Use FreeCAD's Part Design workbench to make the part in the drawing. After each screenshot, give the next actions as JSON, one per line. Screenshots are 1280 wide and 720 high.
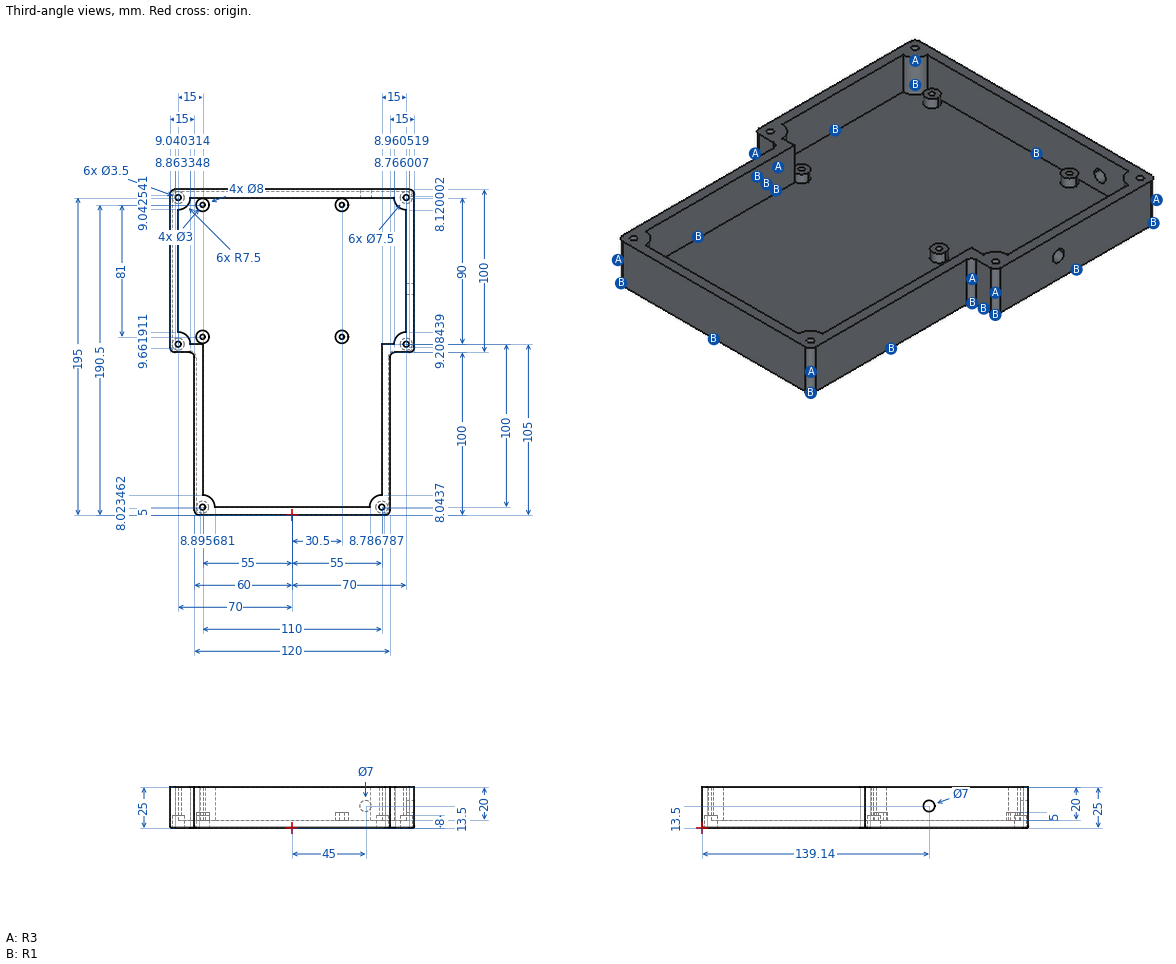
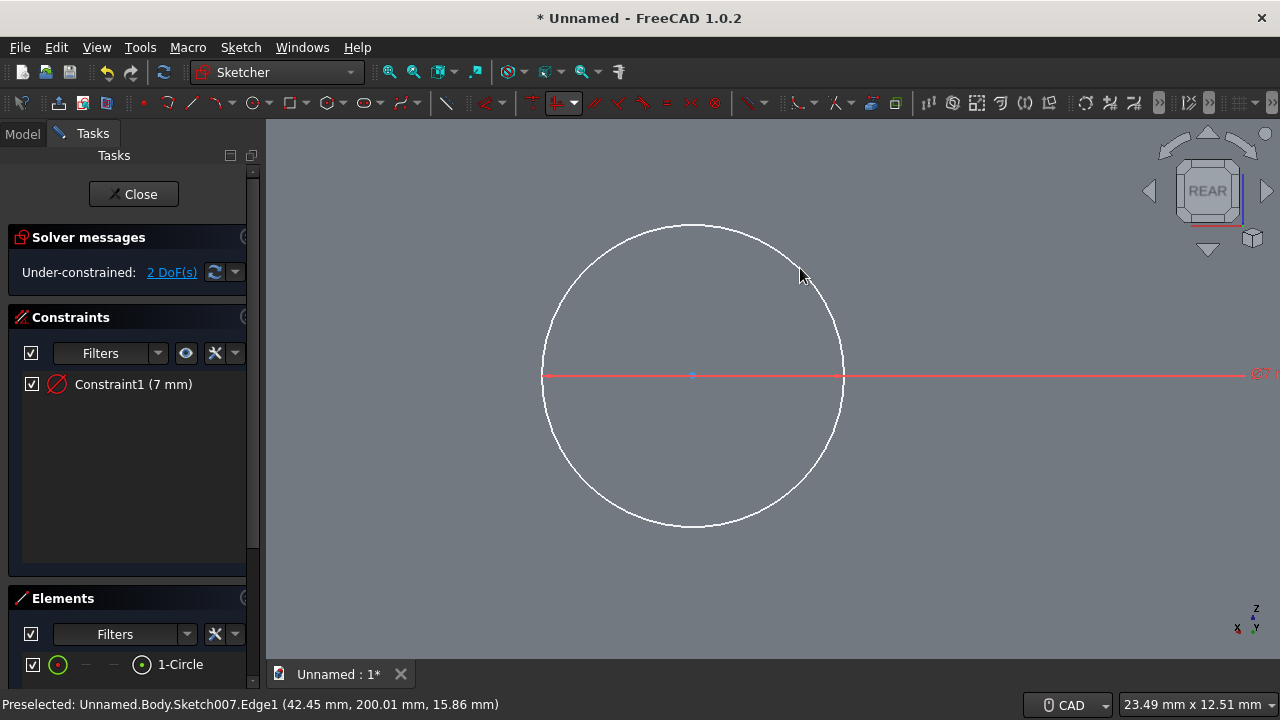
{"action": "key", "text": "d"}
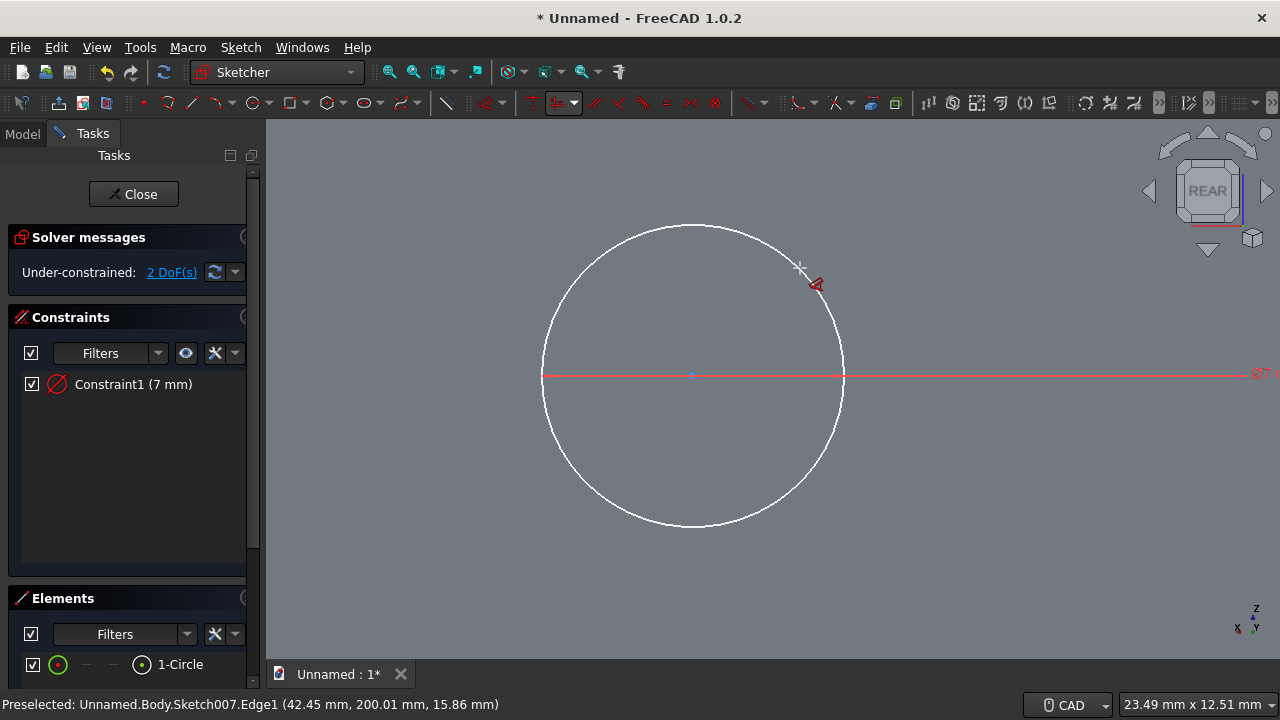
{"action": "left_click", "coordinate": [693, 376]}
{"action": "left_click", "coordinate": [904, 342]}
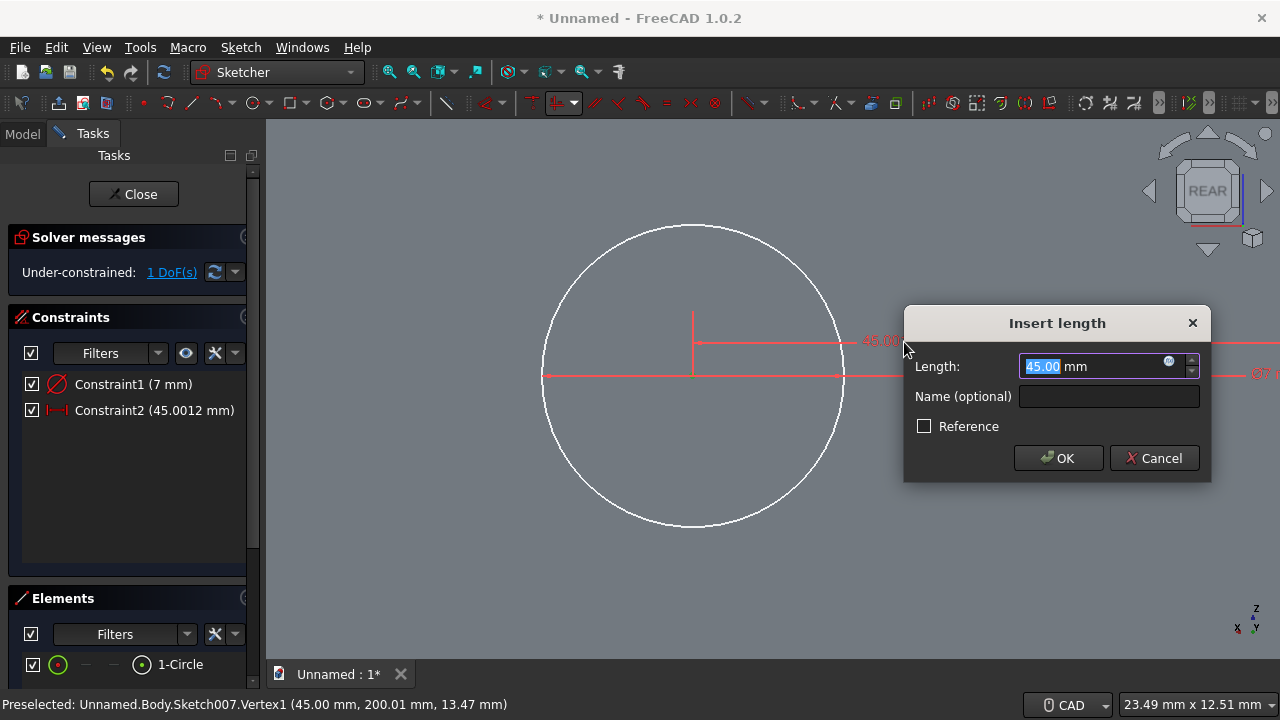
{"action": "type", "text": "45"}
{"action": "key", "text": "Return"}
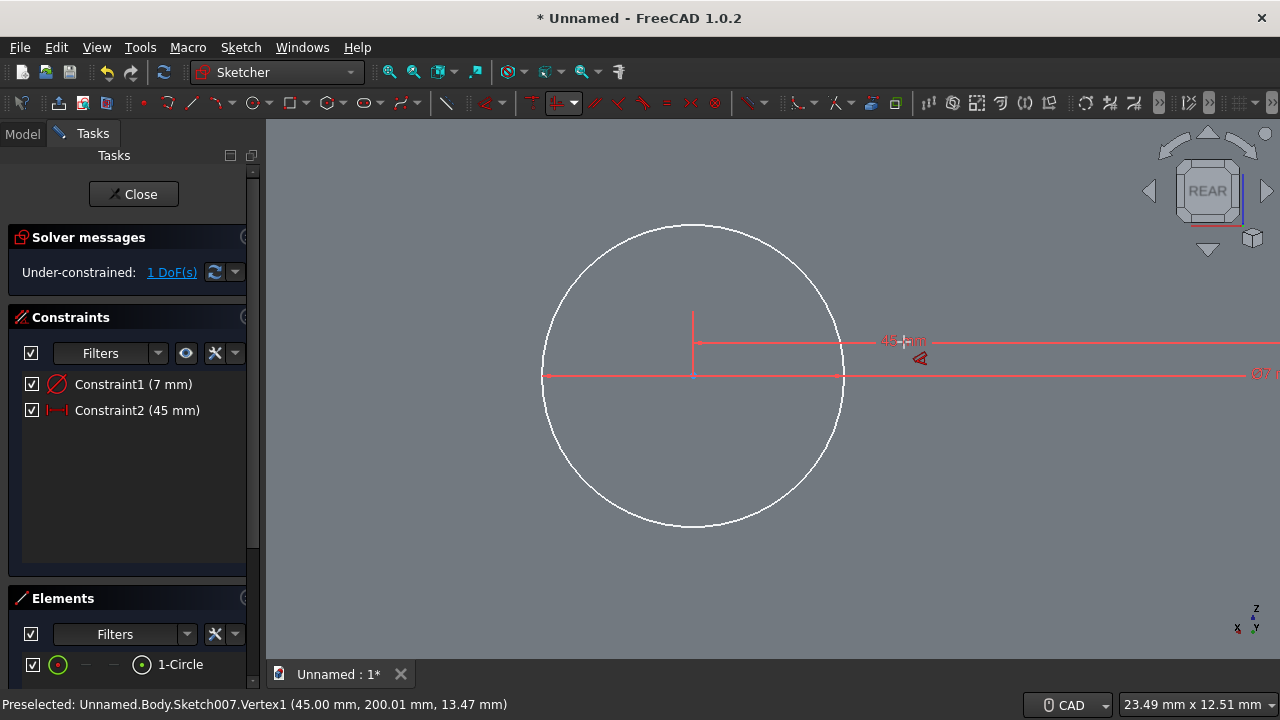
{"action": "left_click", "coordinate": [693, 376]}
{"action": "left_click", "coordinate": [659, 503]}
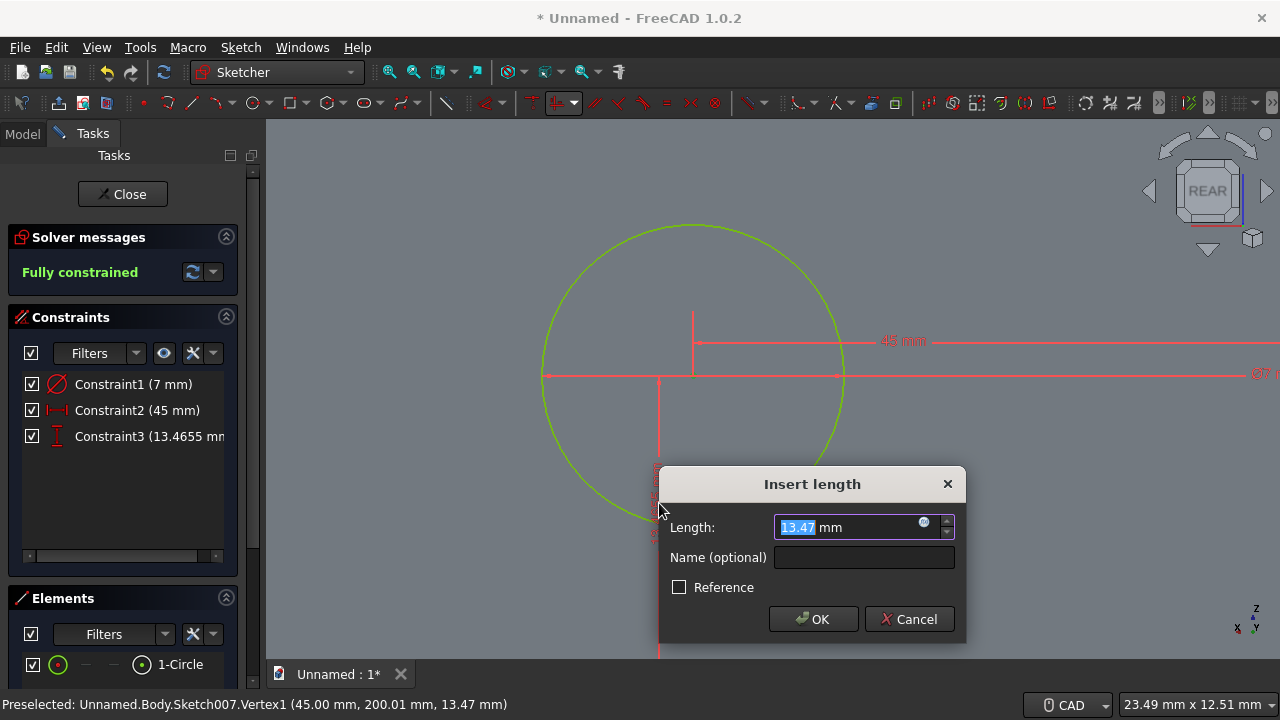
{"action": "type", "text": "13.5"}
{"action": "key", "text": "Return"}
{"action": "key", "text": "Escape"}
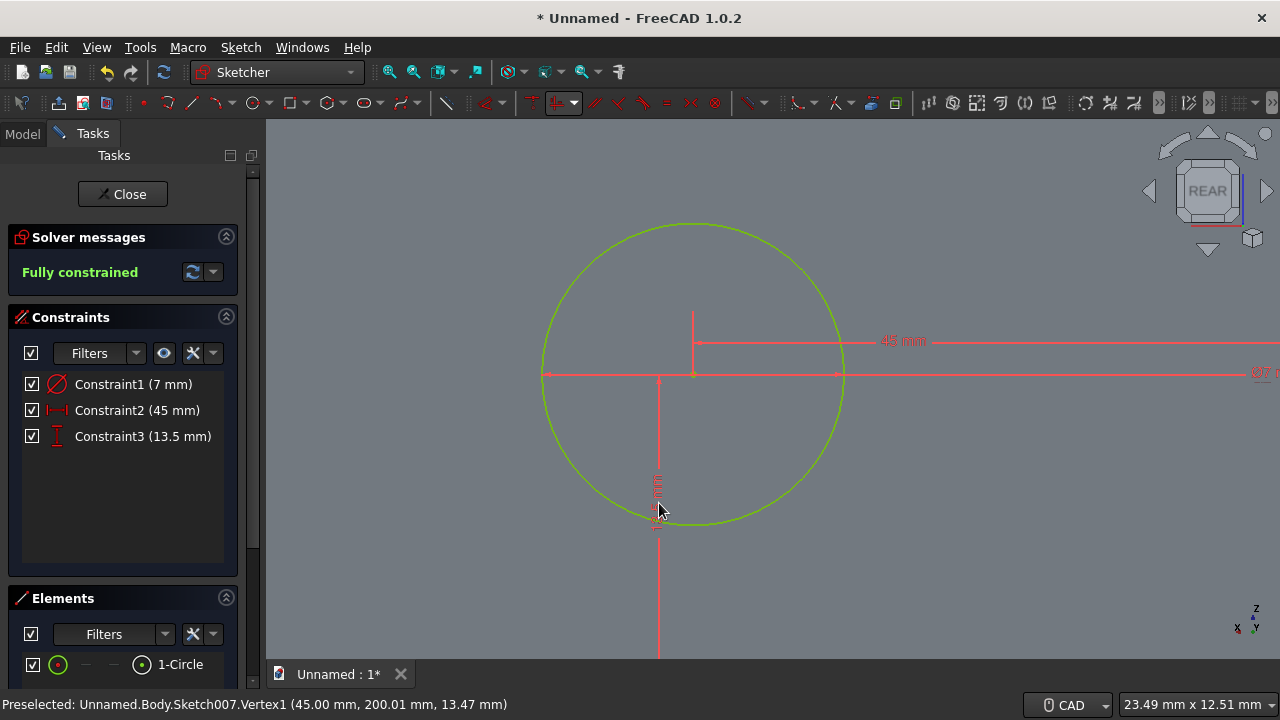
{"action": "left_click", "coordinate": [123, 194]}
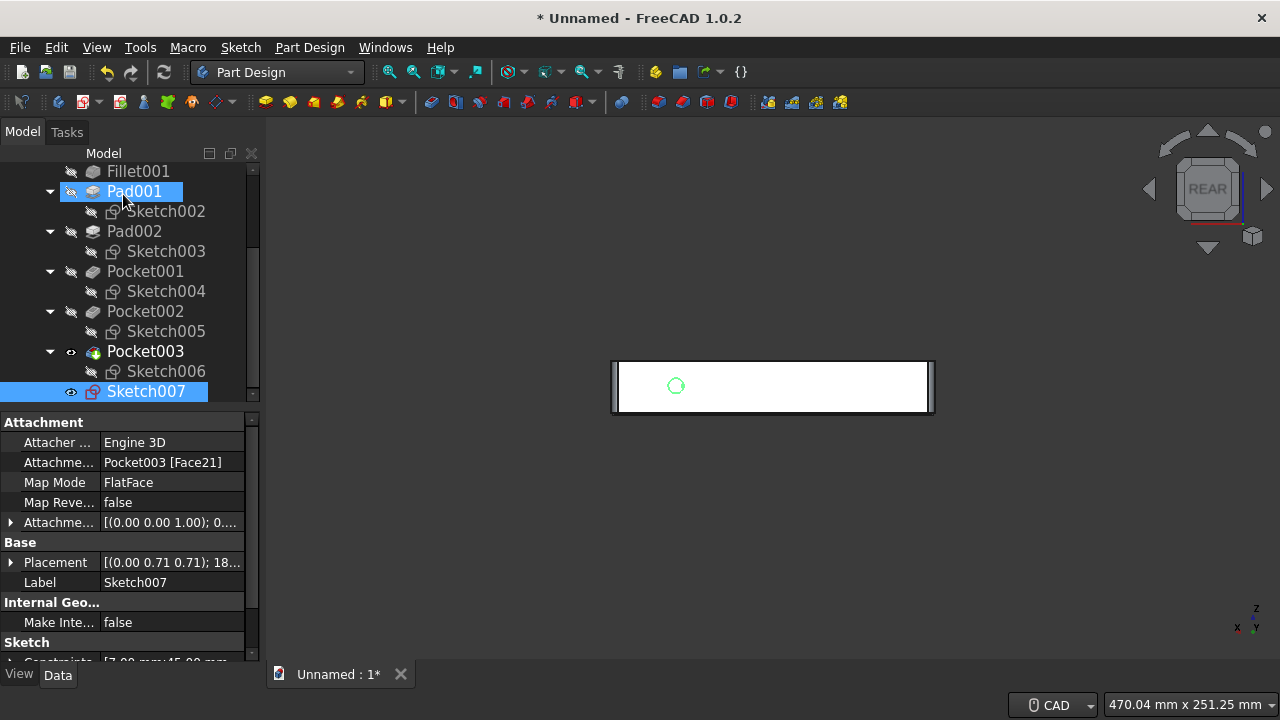
{"action": "left_click", "coordinate": [432, 102]}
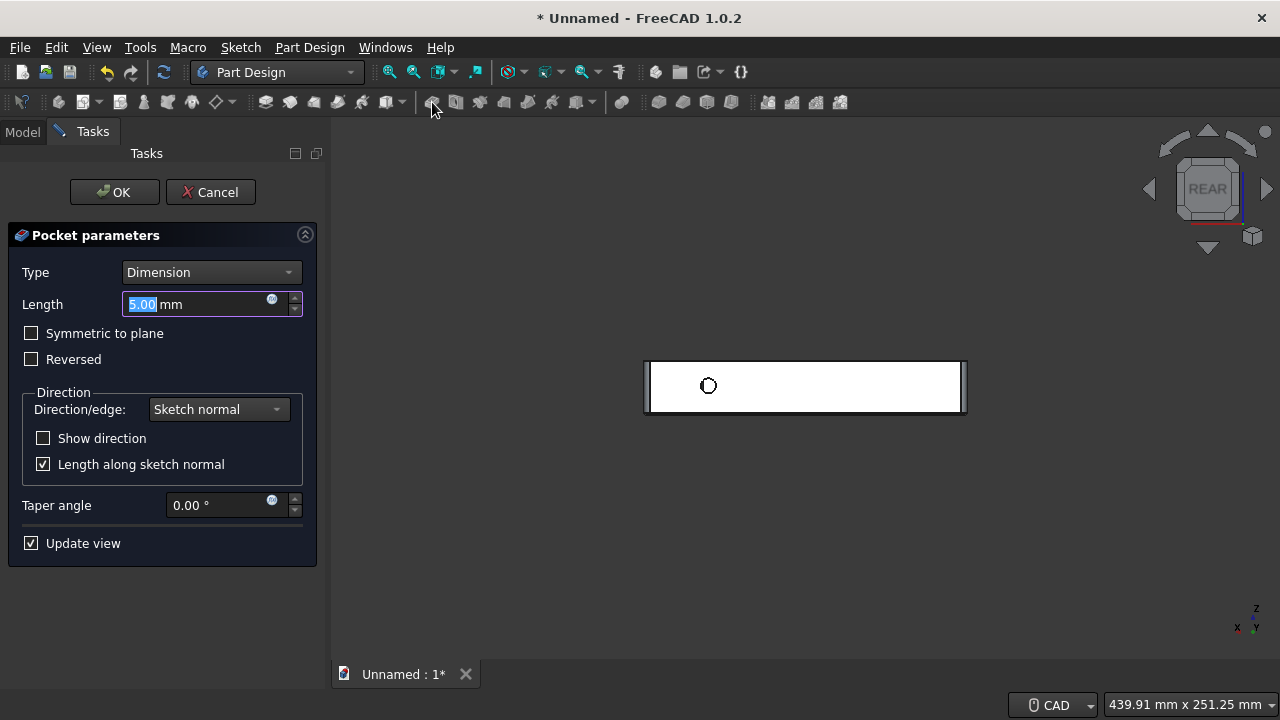
{"action": "left_click", "coordinate": [212, 272]}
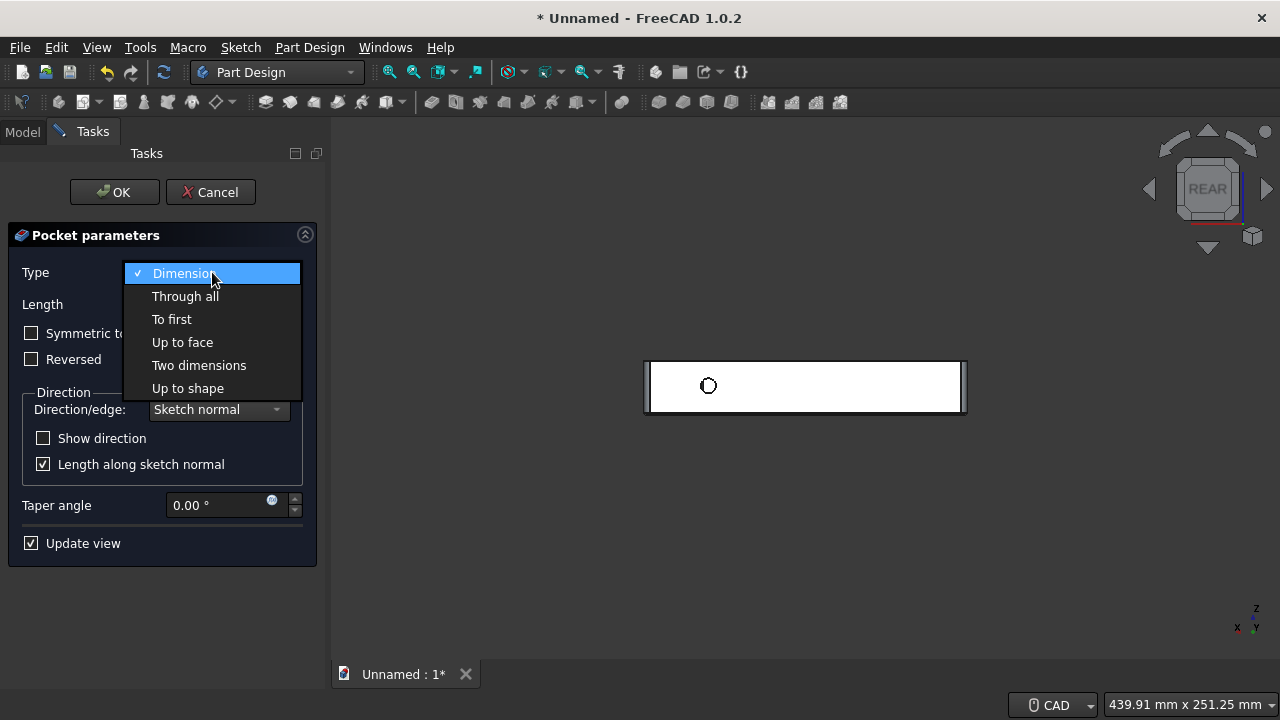
{"action": "left_click", "coordinate": [212, 320]}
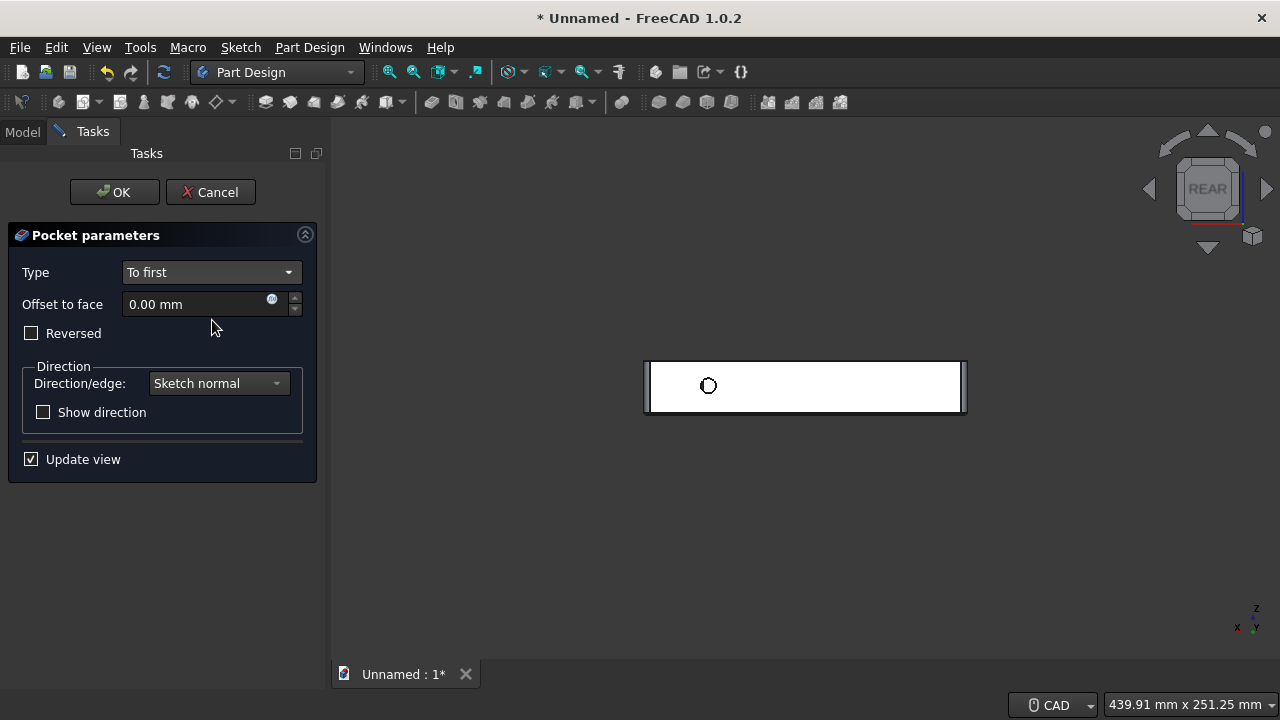
{"action": "left_click", "coordinate": [115, 192]}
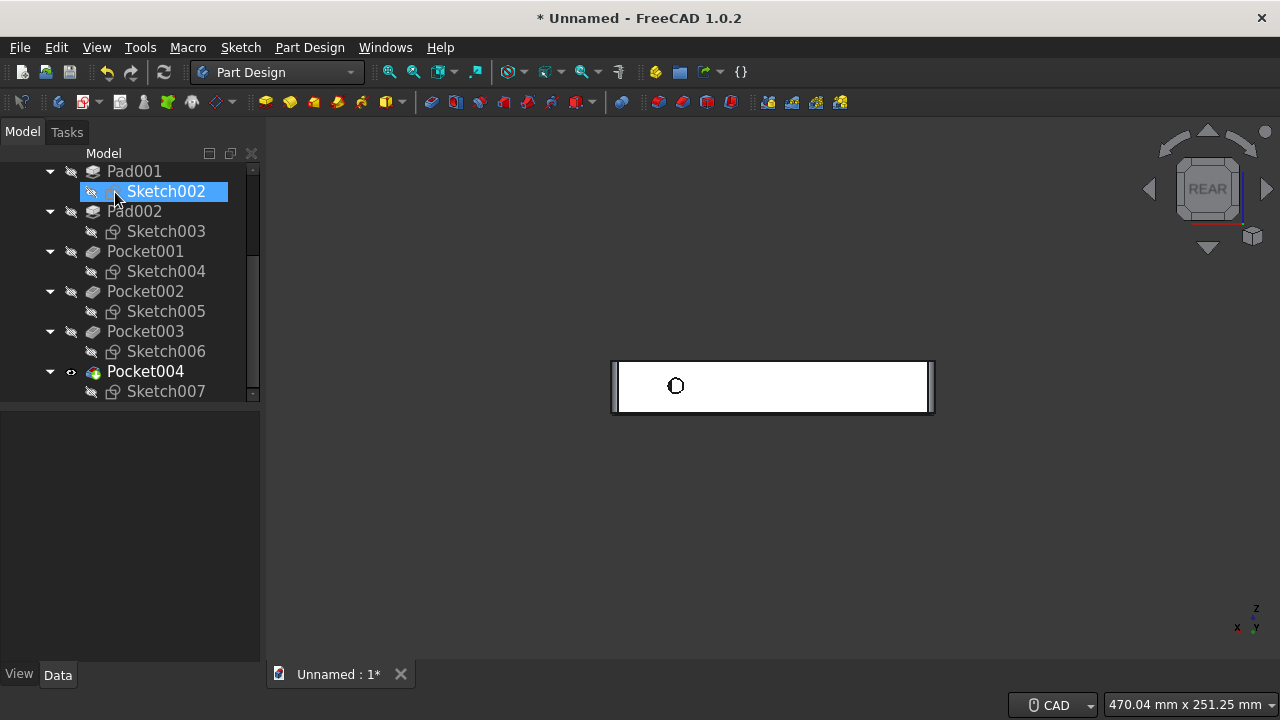
{"action": "key", "text": "0"}